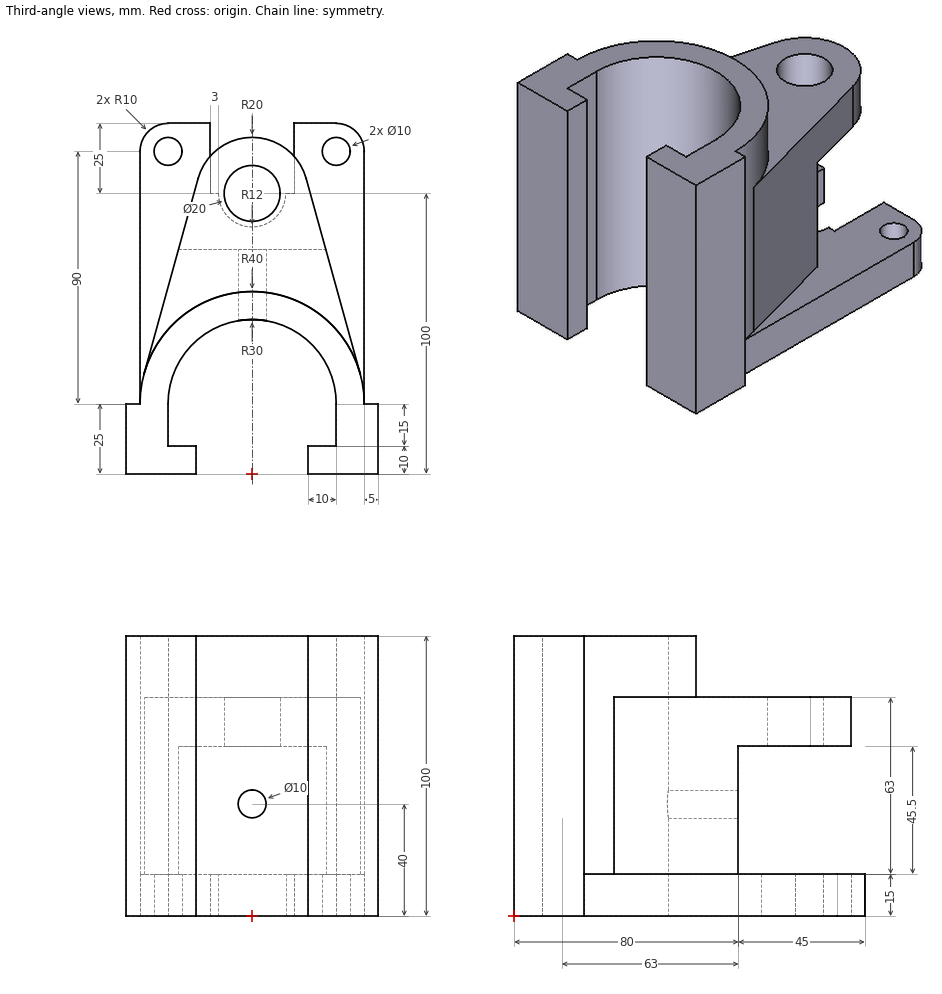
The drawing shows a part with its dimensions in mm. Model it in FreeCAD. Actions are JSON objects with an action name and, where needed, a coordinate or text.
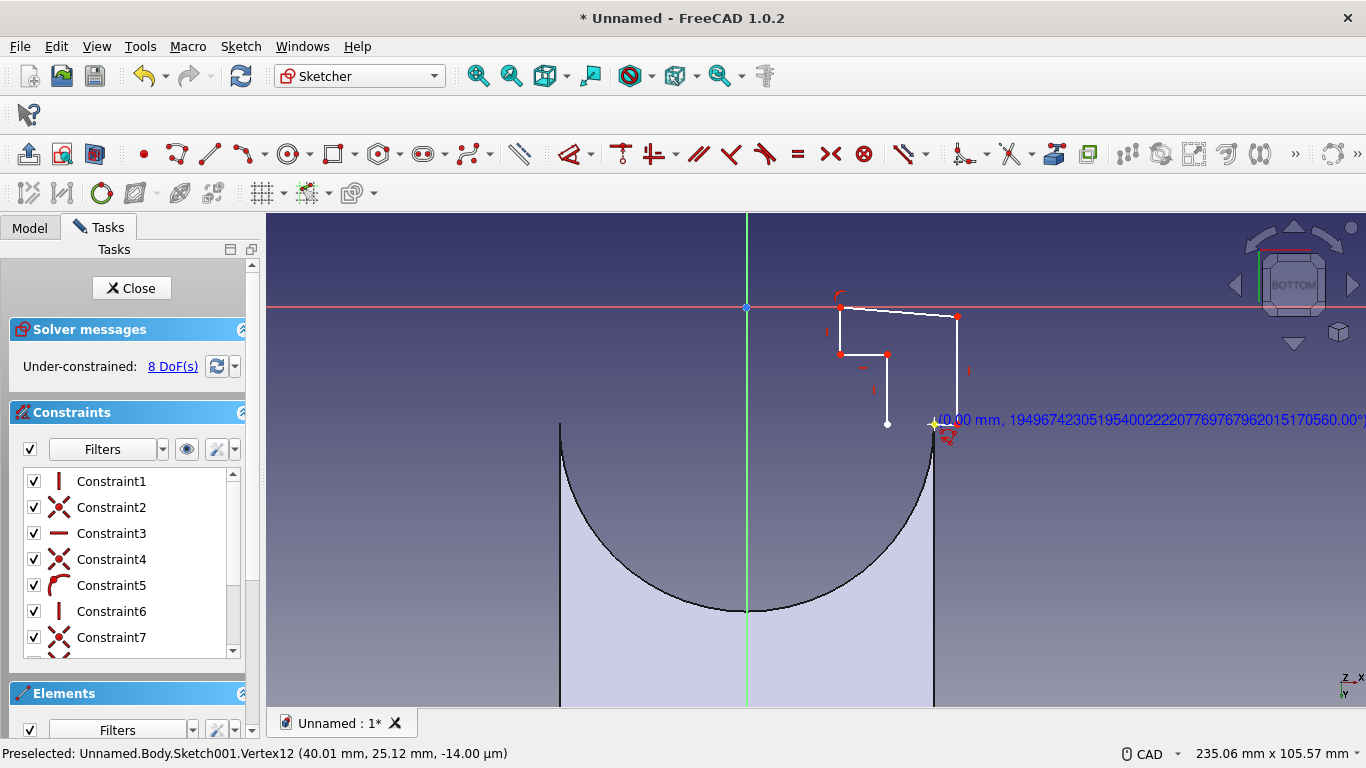
{"action": "left_click", "coordinate": [560, 424]}
{"action": "left_click", "coordinate": [536, 424]}
{"action": "left_click", "coordinate": [536, 307]}
{"action": "left_click", "coordinate": [653, 316]}
{"action": "left_click", "coordinate": [653, 354]}
{"action": "left_click", "coordinate": [606, 354]}
{"action": "left_click", "coordinate": [606, 424]}
{"action": "right_click", "coordinate": [606, 424]}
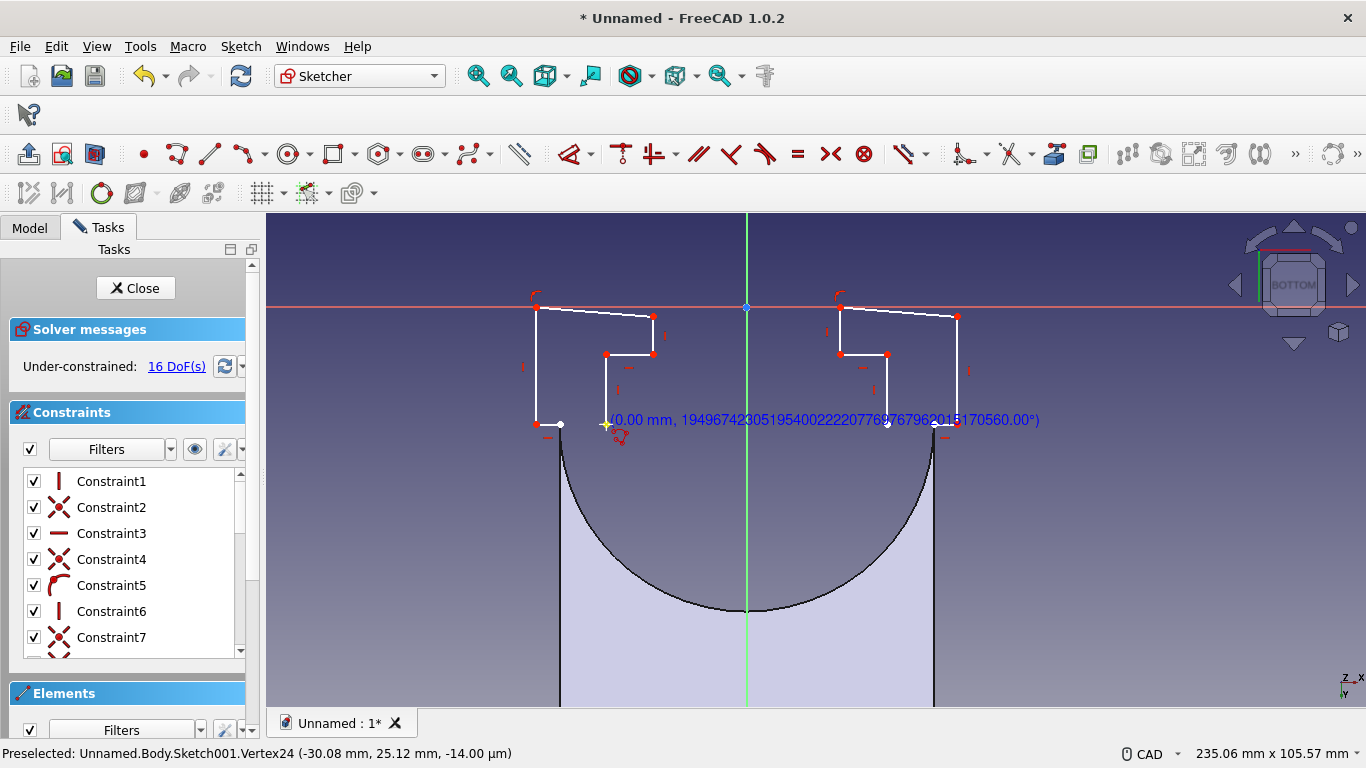
{"action": "key", "text": "g 3 a"}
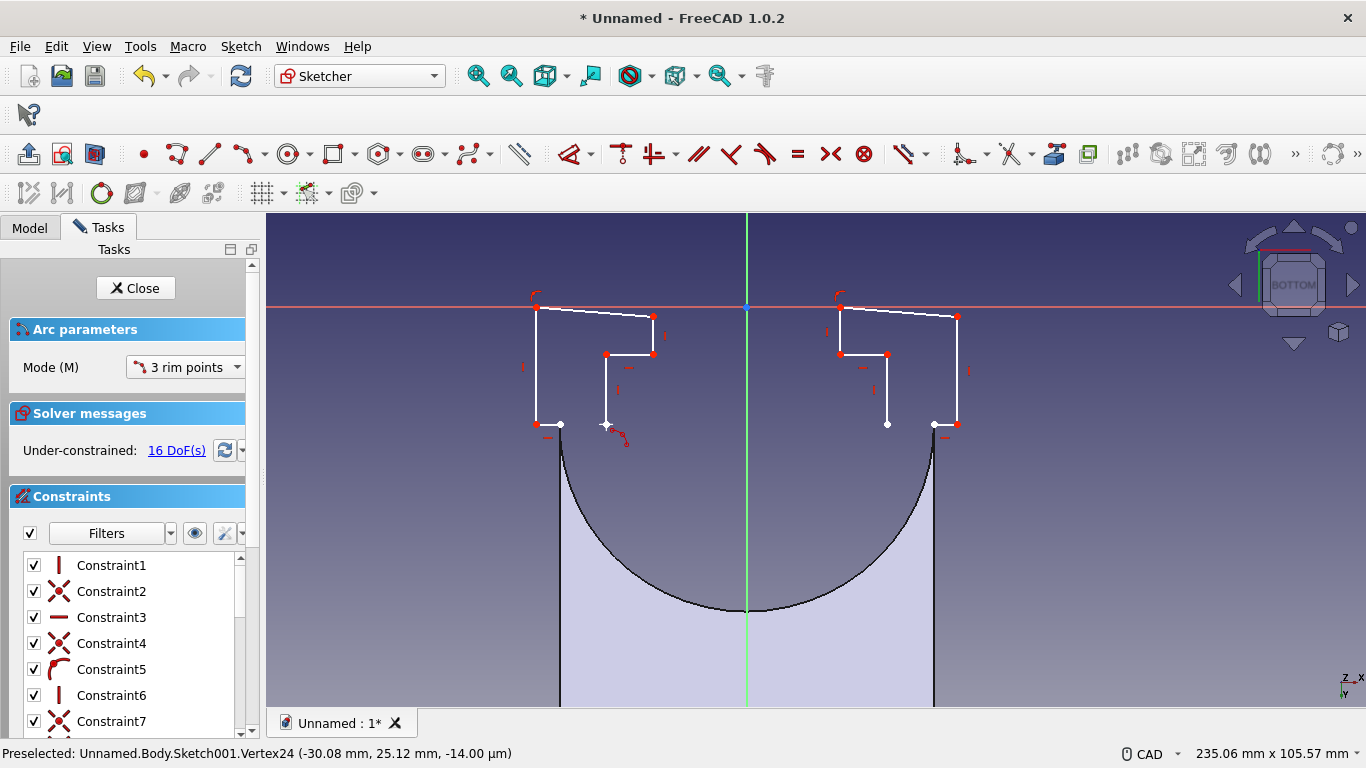
{"action": "scroll", "coordinate": [934, 424], "scroll_direction": "up", "scroll_amount": 2}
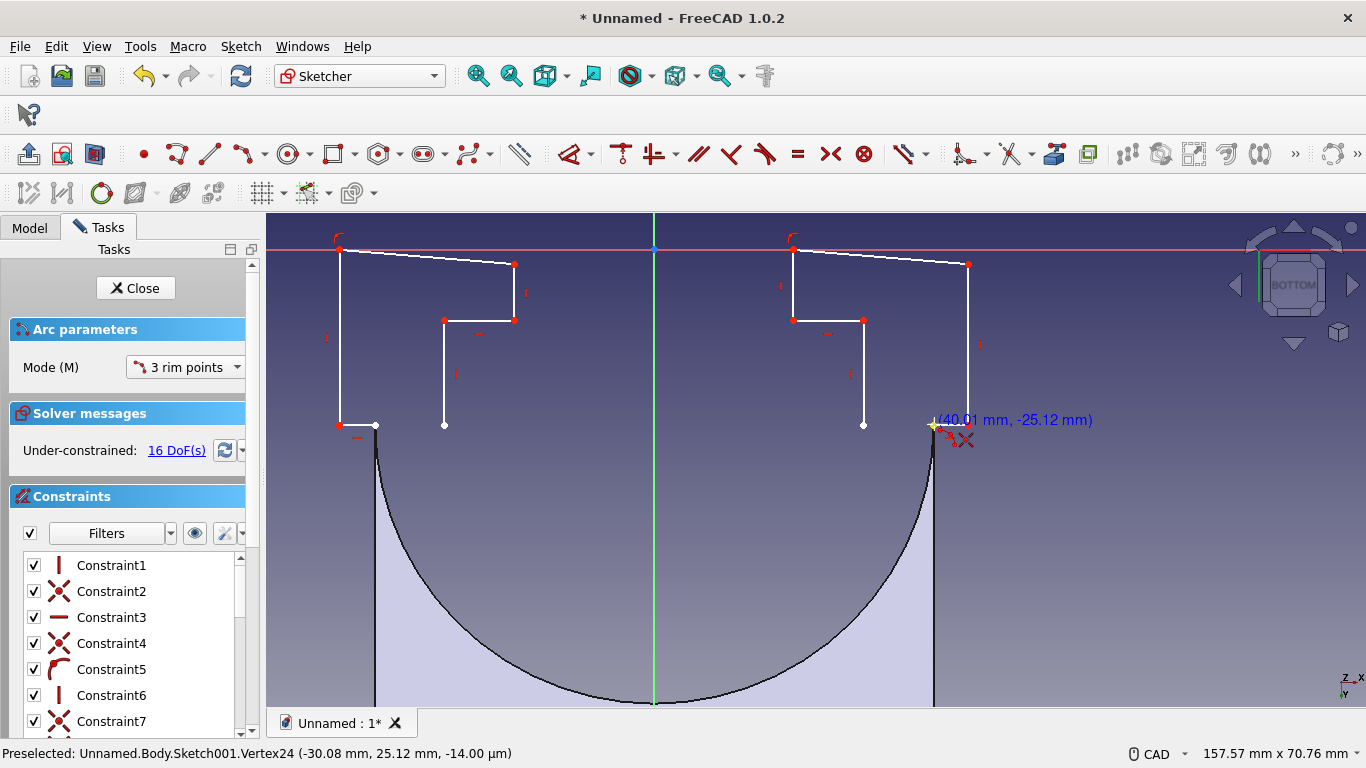
{"action": "left_click", "coordinate": [934, 425]}
{"action": "left_click", "coordinate": [376, 425]}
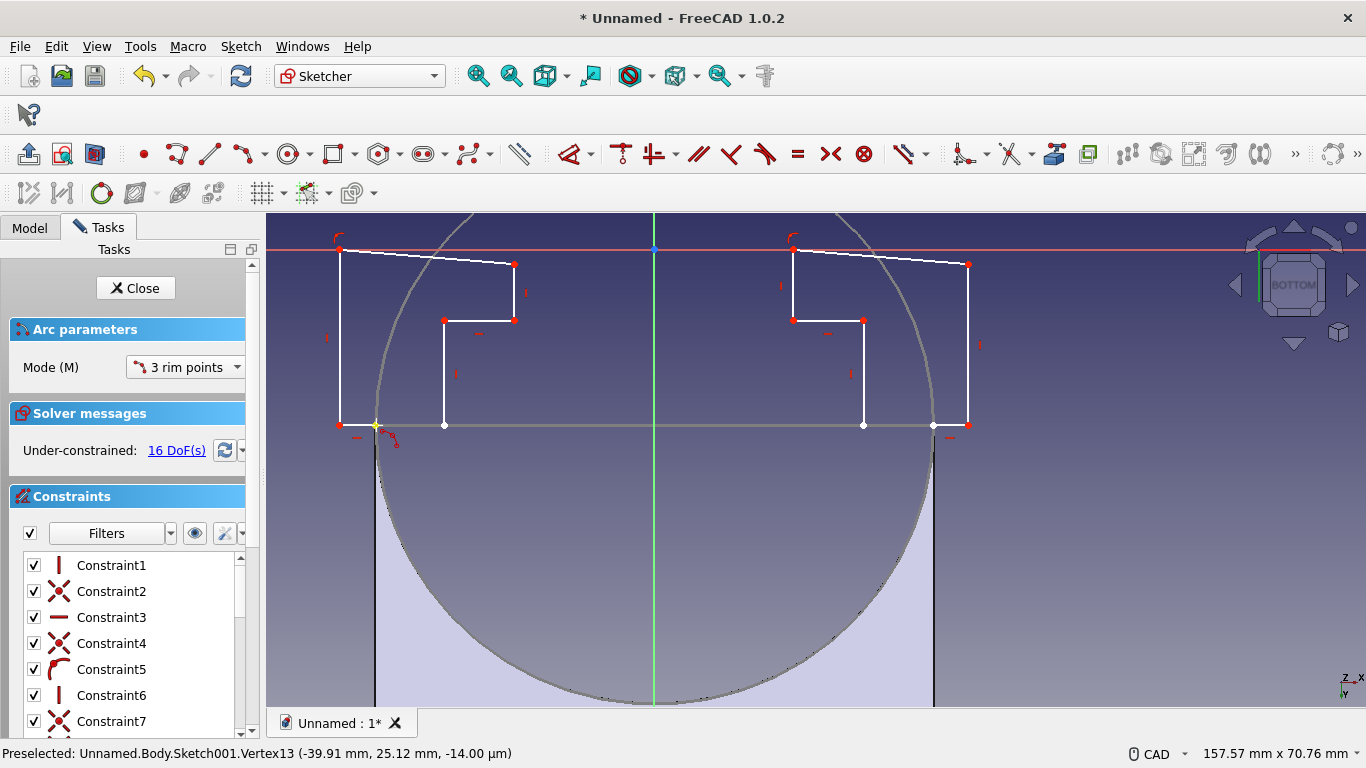
{"action": "scroll", "coordinate": [937, 426], "scroll_direction": "down", "scroll_amount": 2}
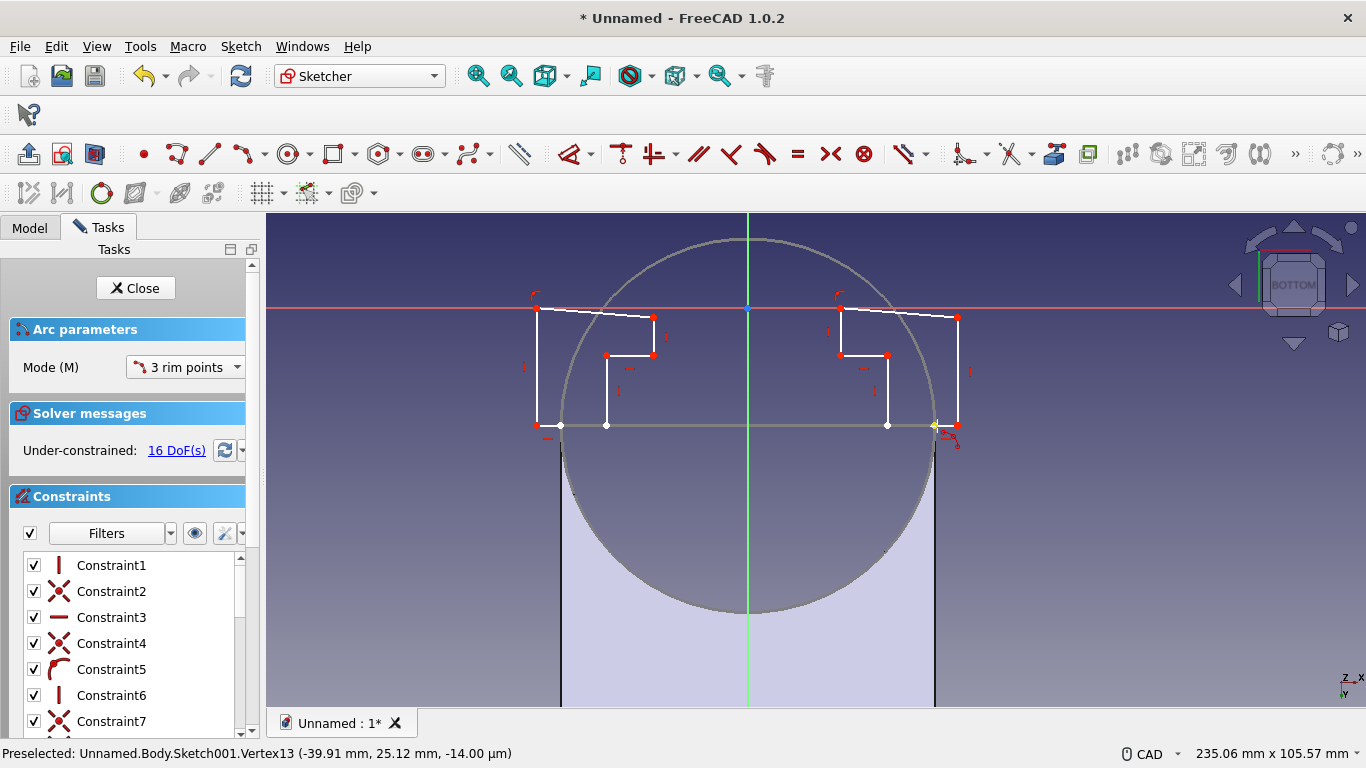
{"action": "left_click", "coordinate": [690, 603]}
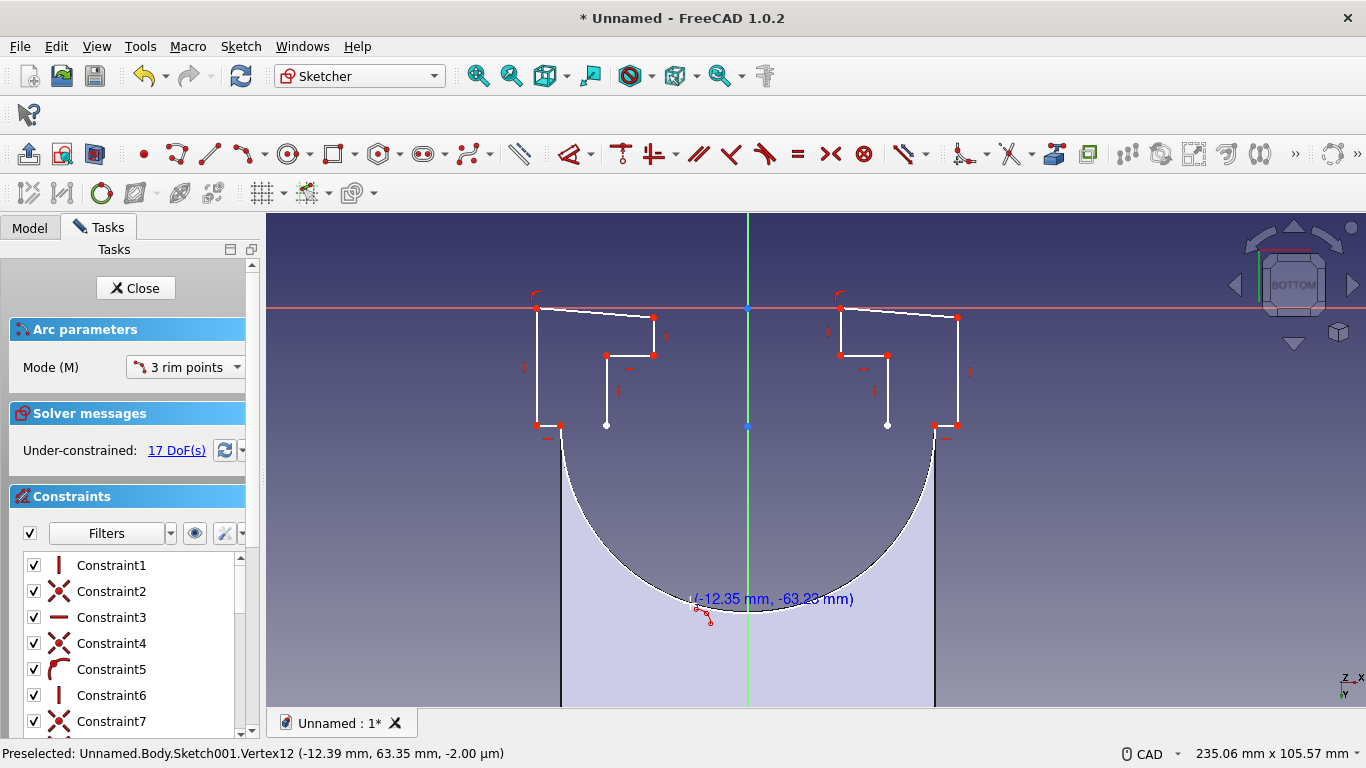
{"action": "left_click", "coordinate": [607, 426]}
{"action": "left_click", "coordinate": [888, 426]}
{"action": "left_click", "coordinate": [704, 559]}
{"action": "key", "text": "Escape"}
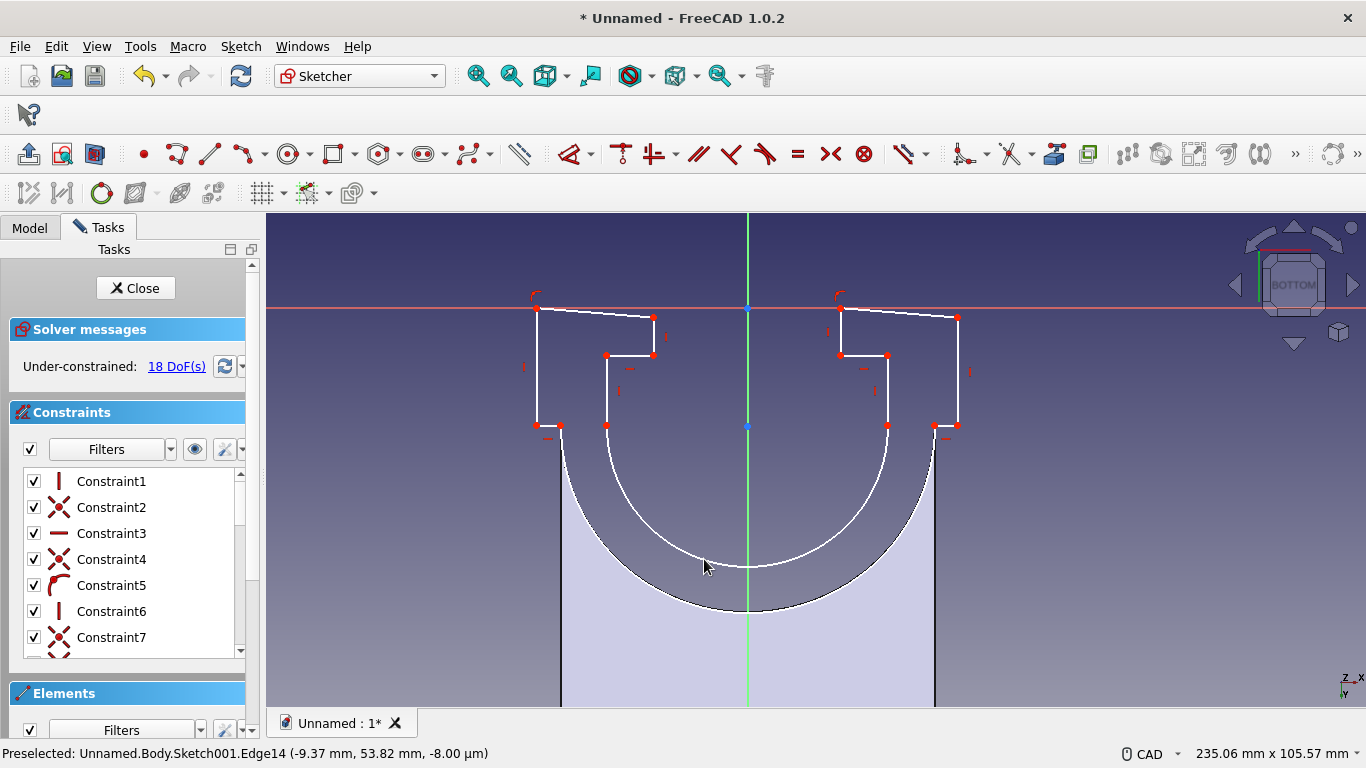
{"action": "left_click", "coordinate": [888, 405]}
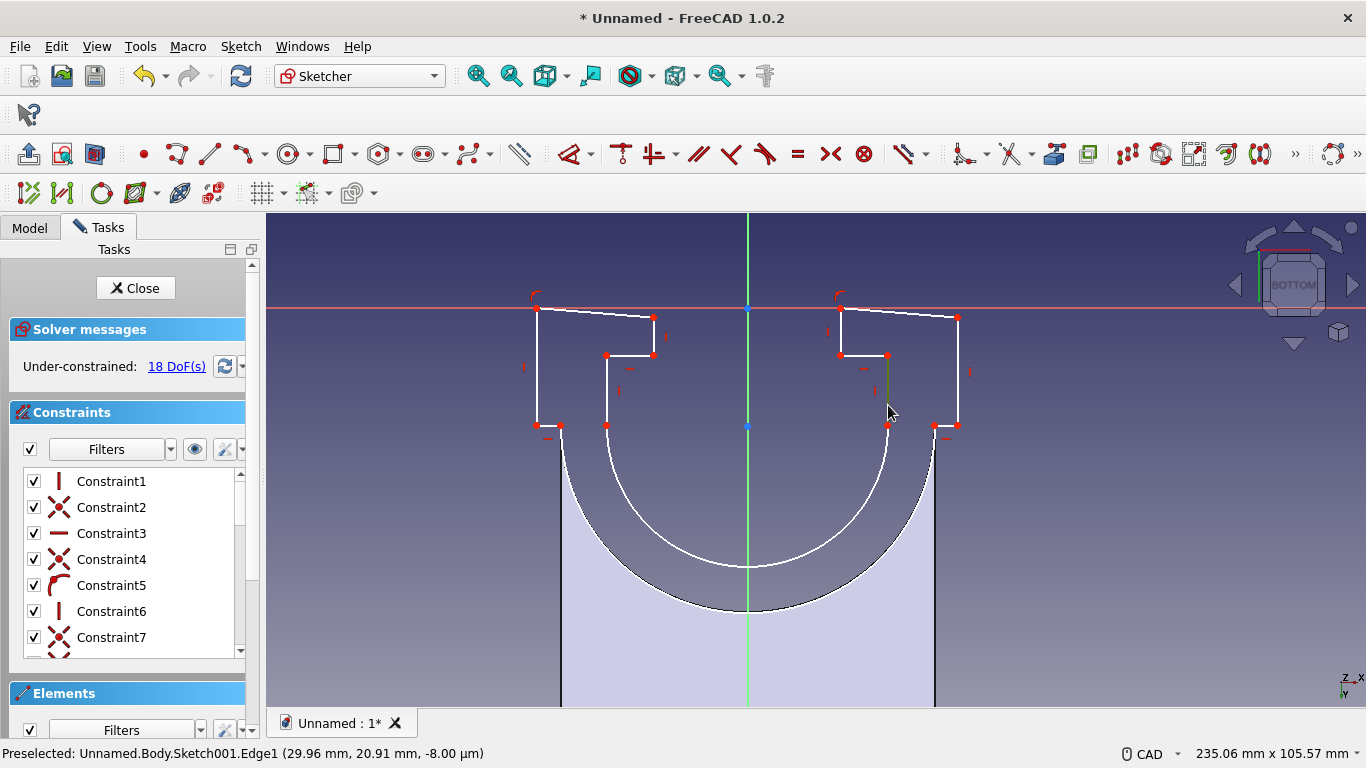
{"action": "left_click", "coordinate": [665, 540]}